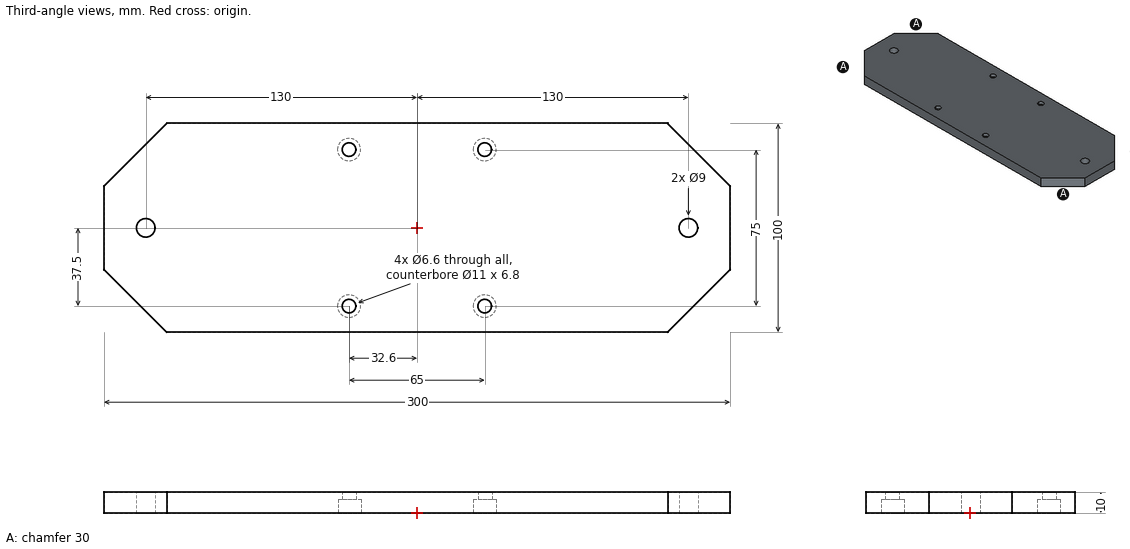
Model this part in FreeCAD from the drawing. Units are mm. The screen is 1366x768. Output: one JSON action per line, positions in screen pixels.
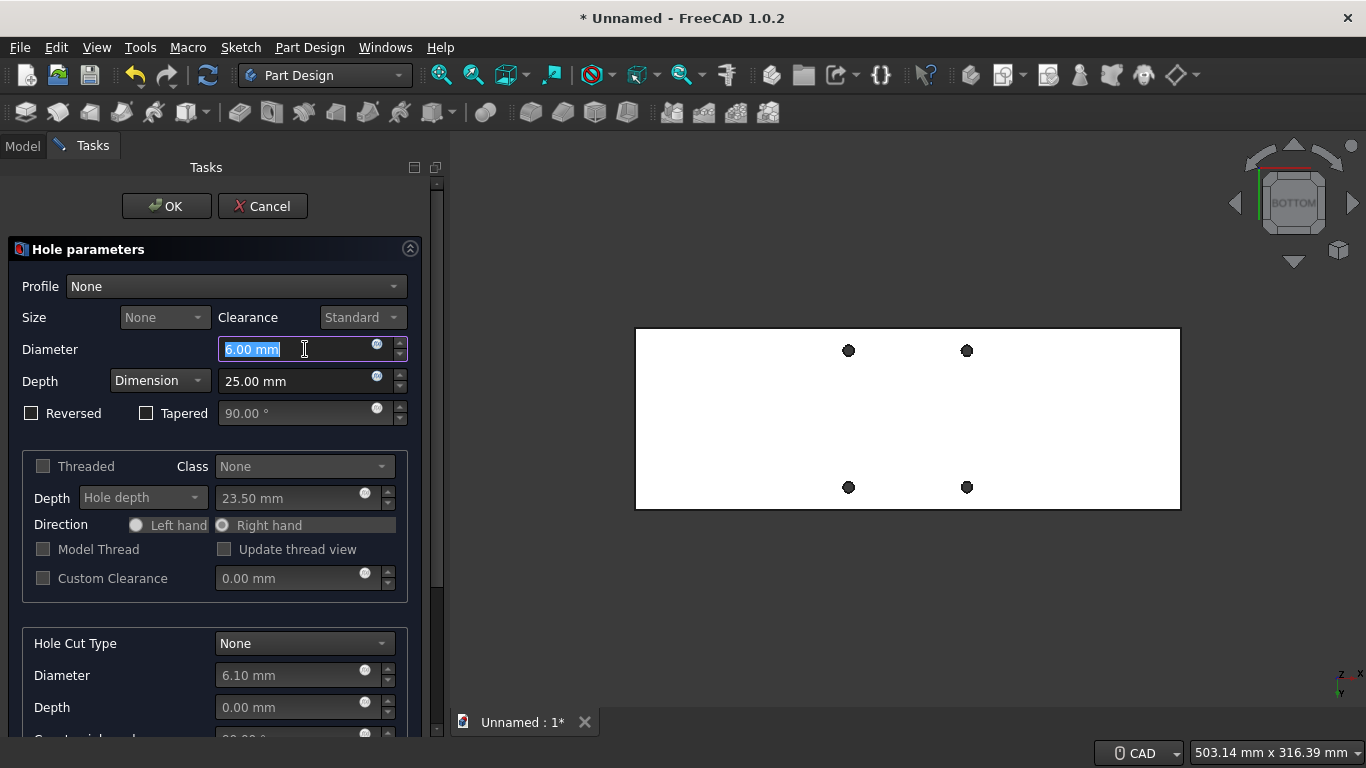
{"action": "type", "text": "6.6"}
{"action": "key", "text": "Tab"}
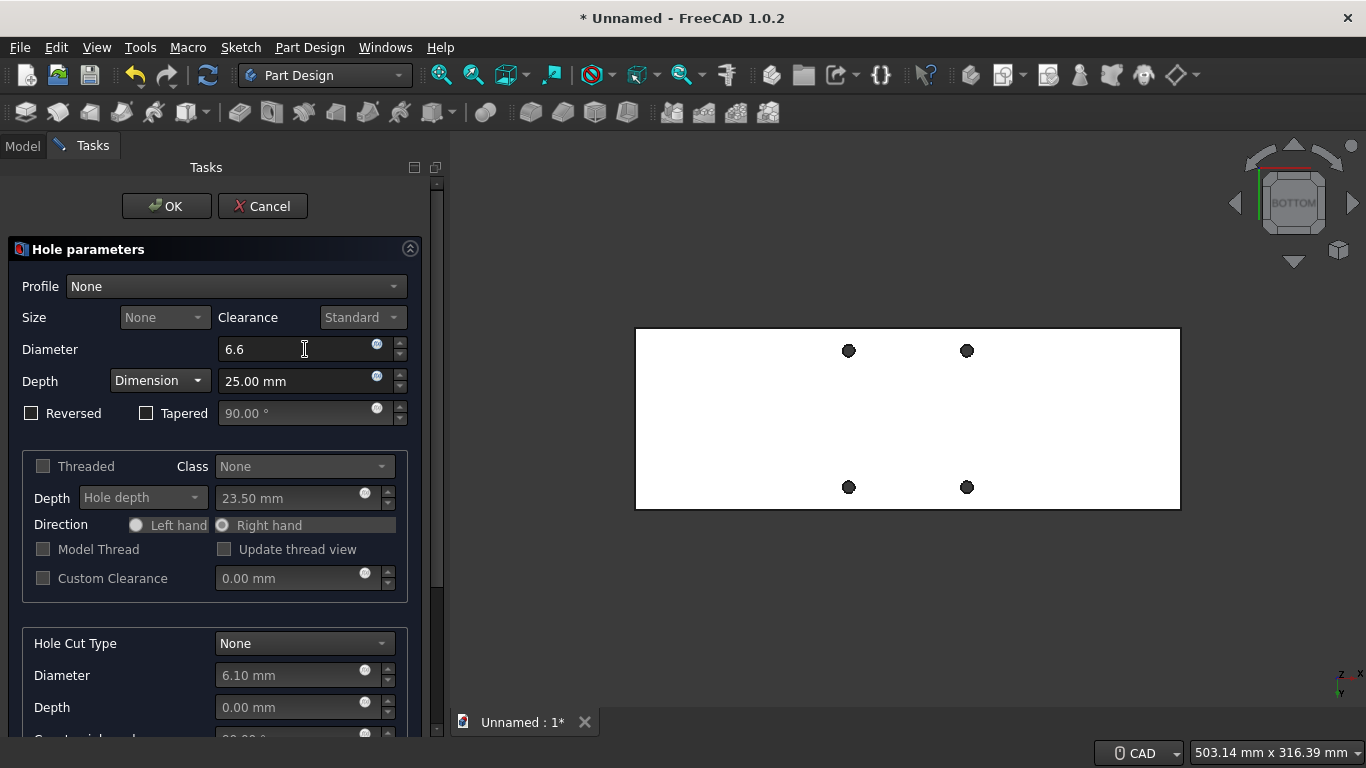
{"action": "left_click", "coordinate": [161, 380]}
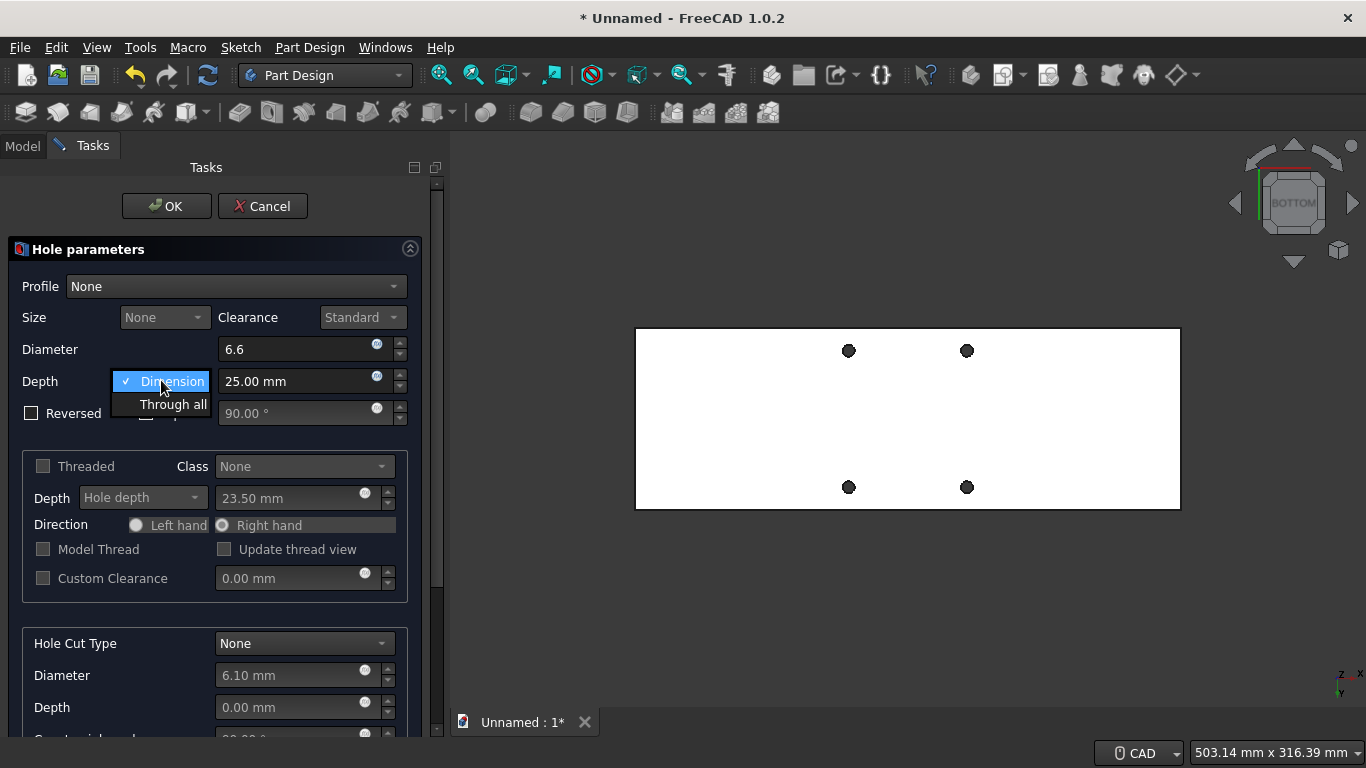
{"action": "left_click", "coordinate": [160, 404]}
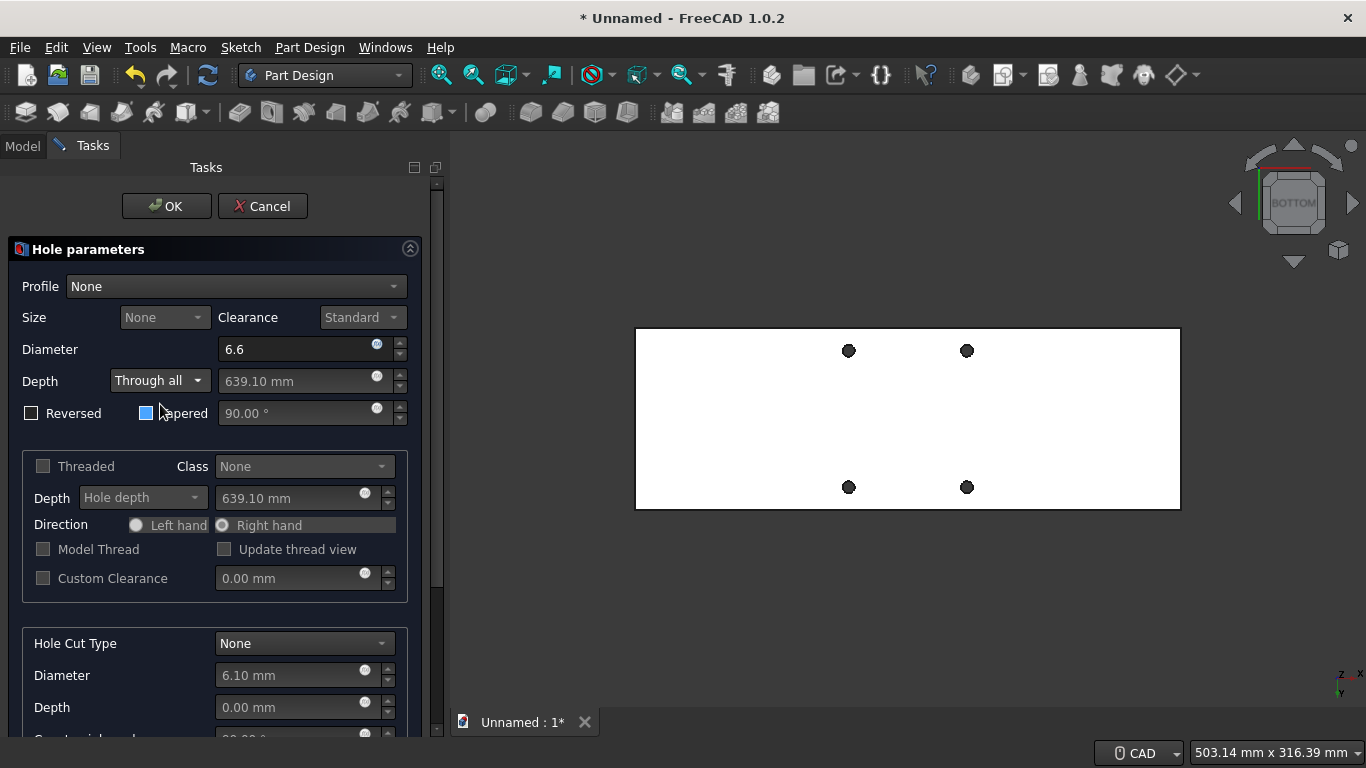
{"action": "left_click", "coordinate": [306, 644]}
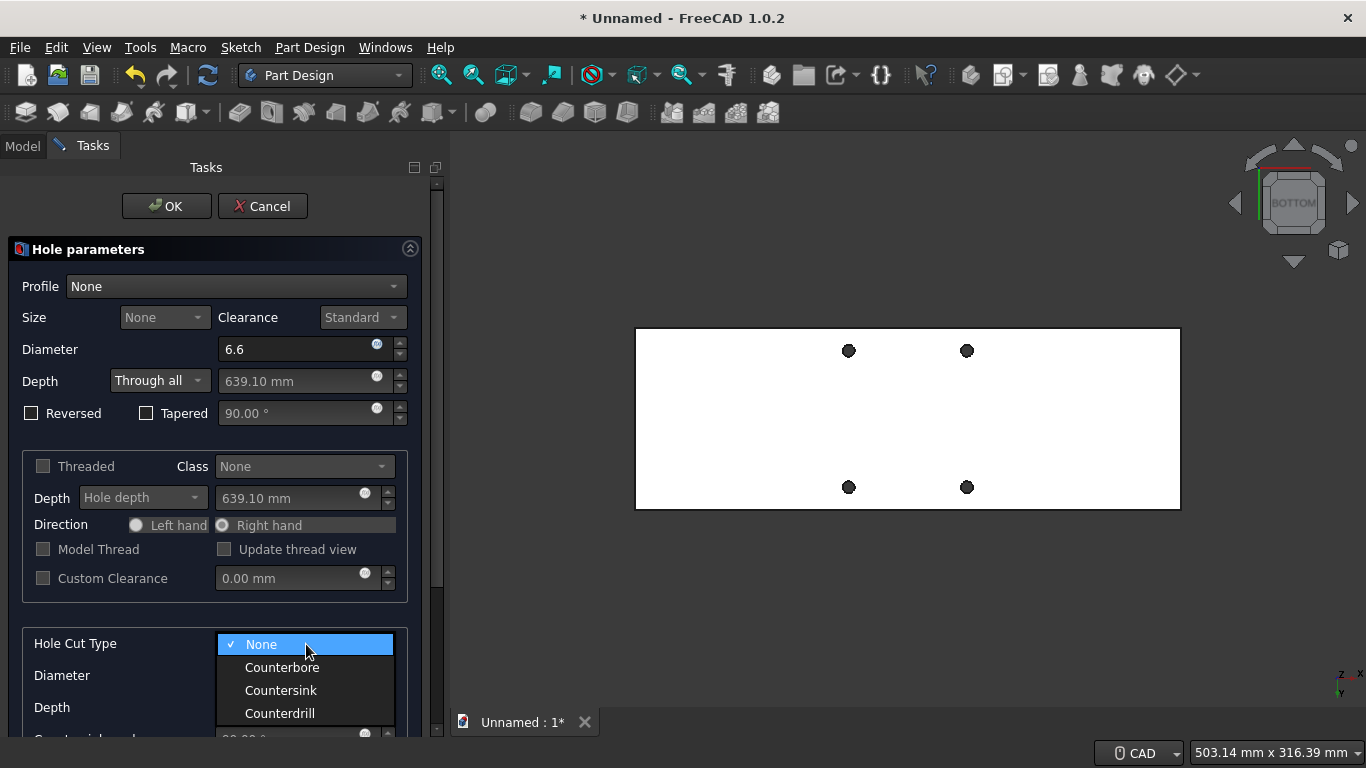
{"action": "left_click", "coordinate": [304, 668]}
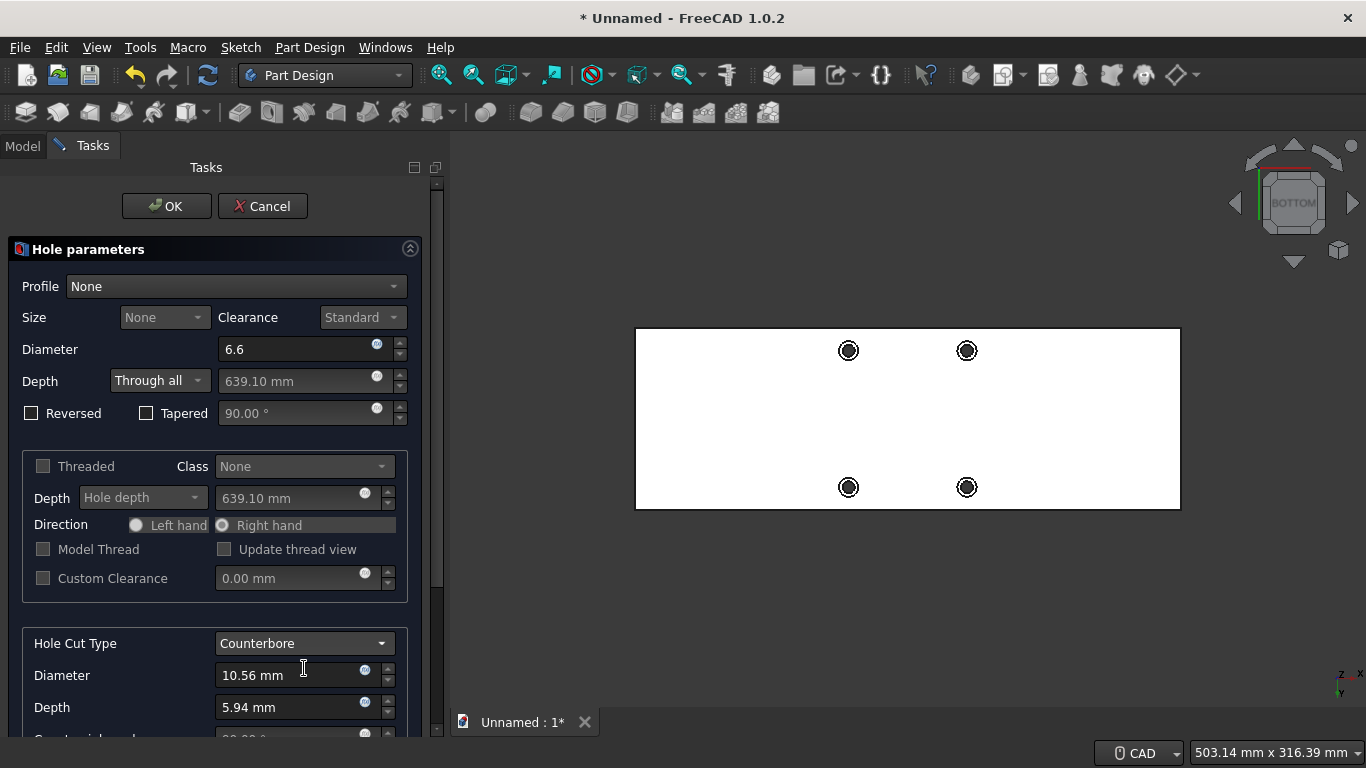
{"action": "triple_click", "coordinate": [298, 675]}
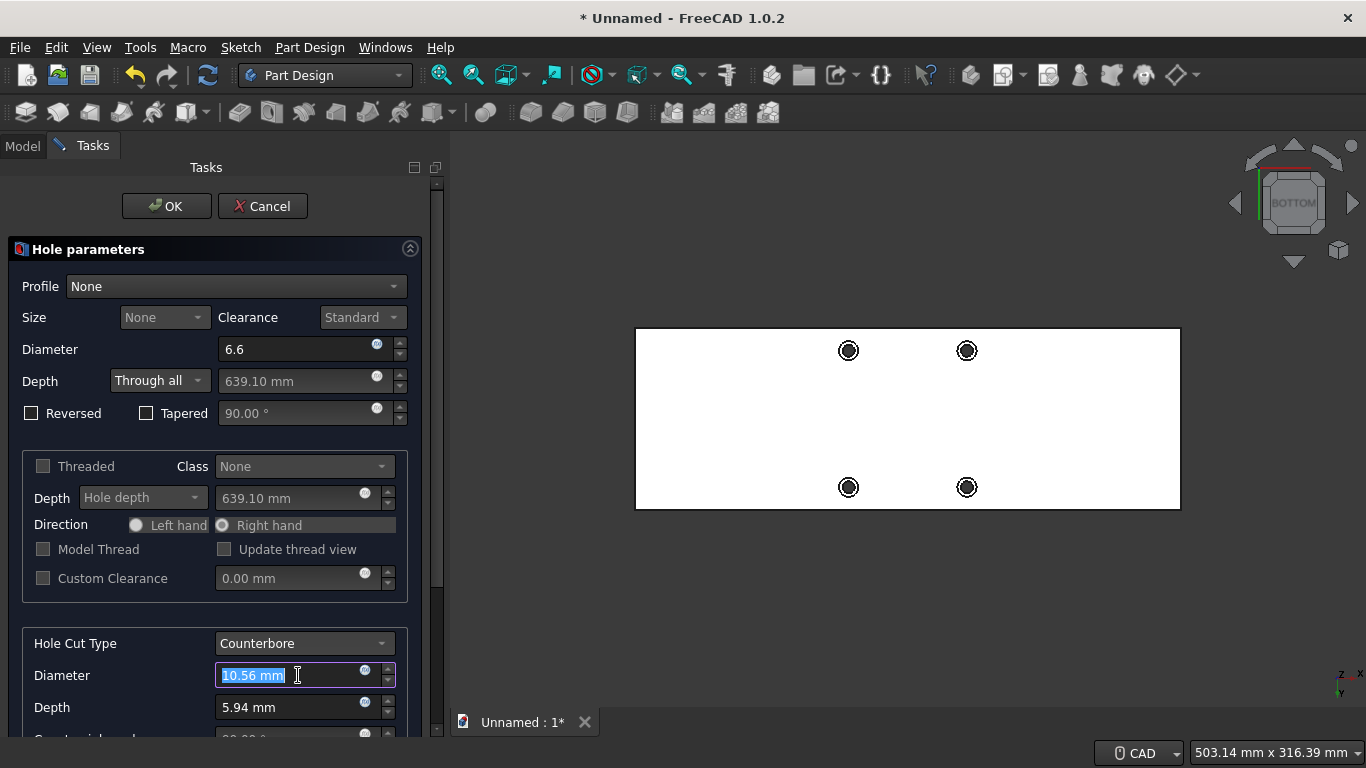
{"action": "type", "text": "11"}
{"action": "key", "text": "Tab"}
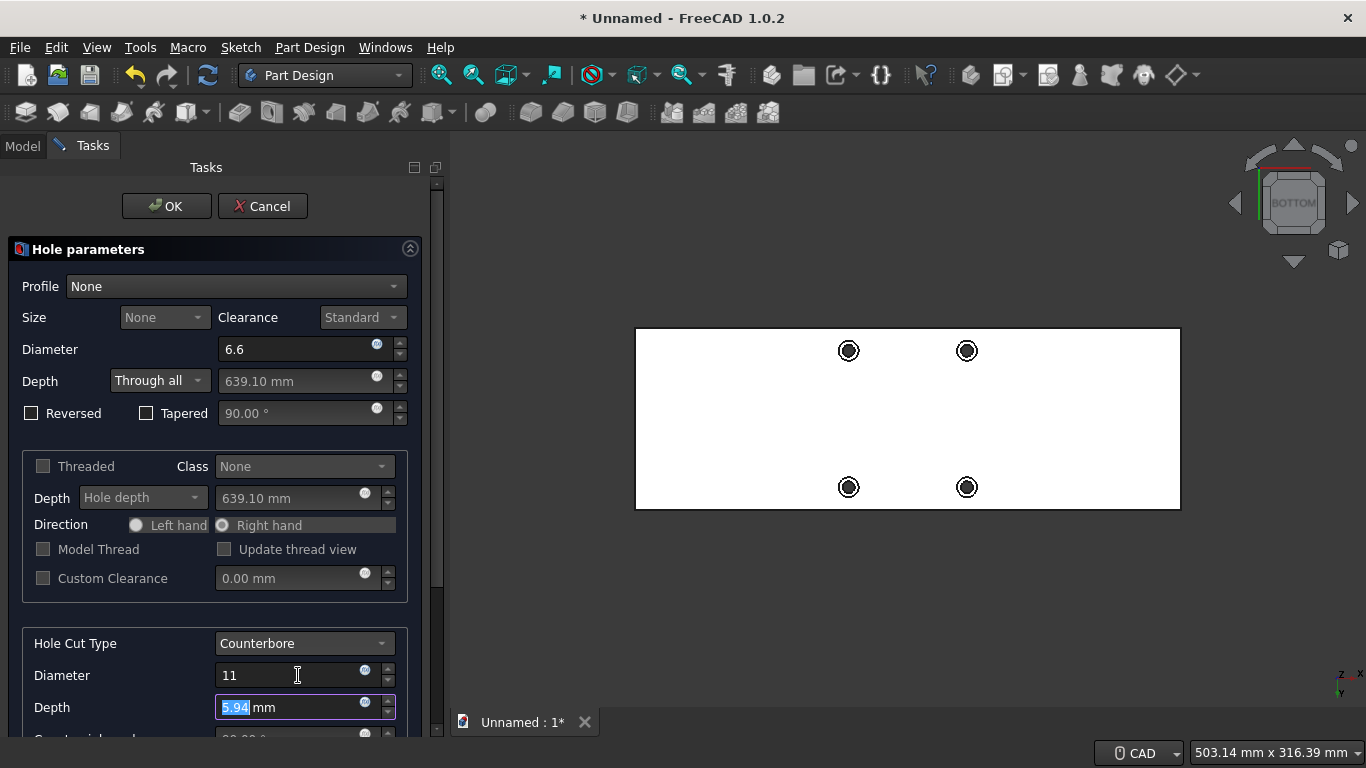
{"action": "type", "text": "6.8"}
{"action": "key", "text": "Tab"}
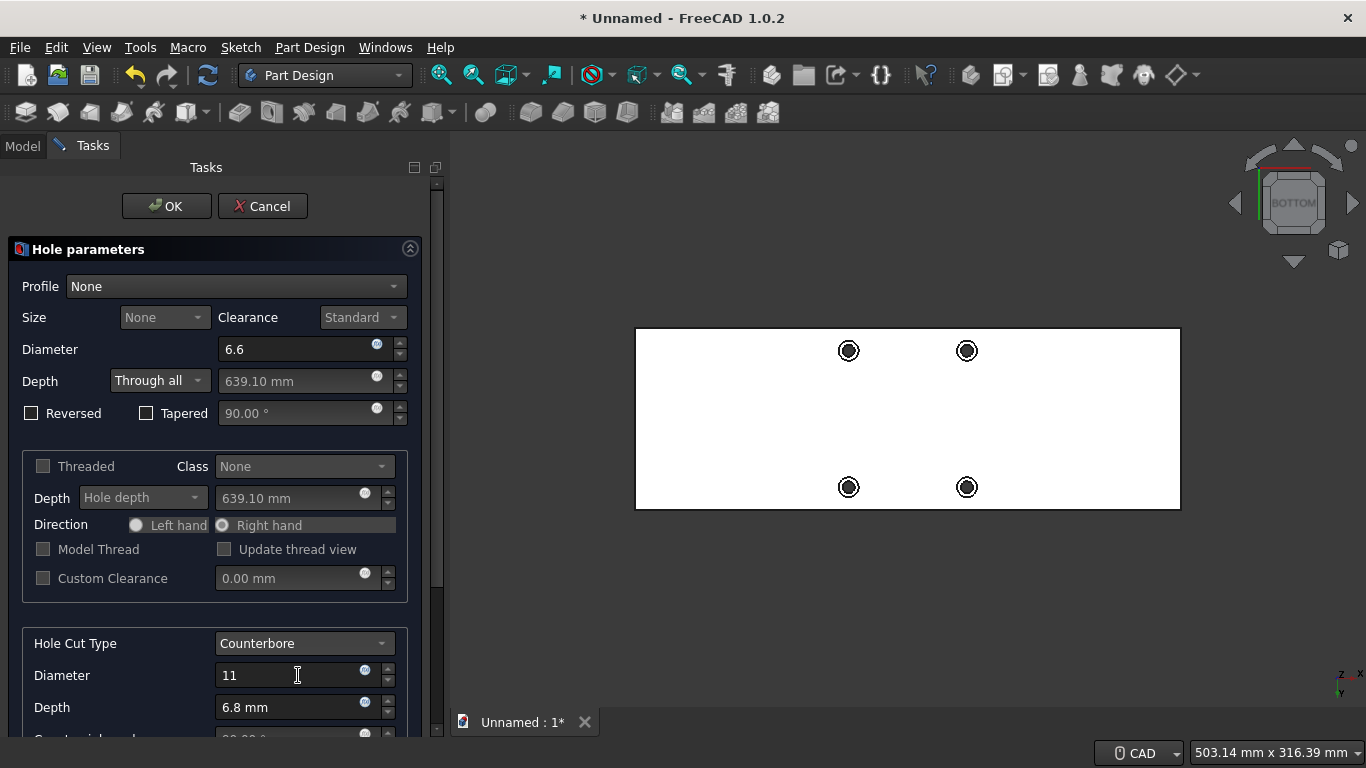
{"action": "left_click", "coordinate": [167, 206]}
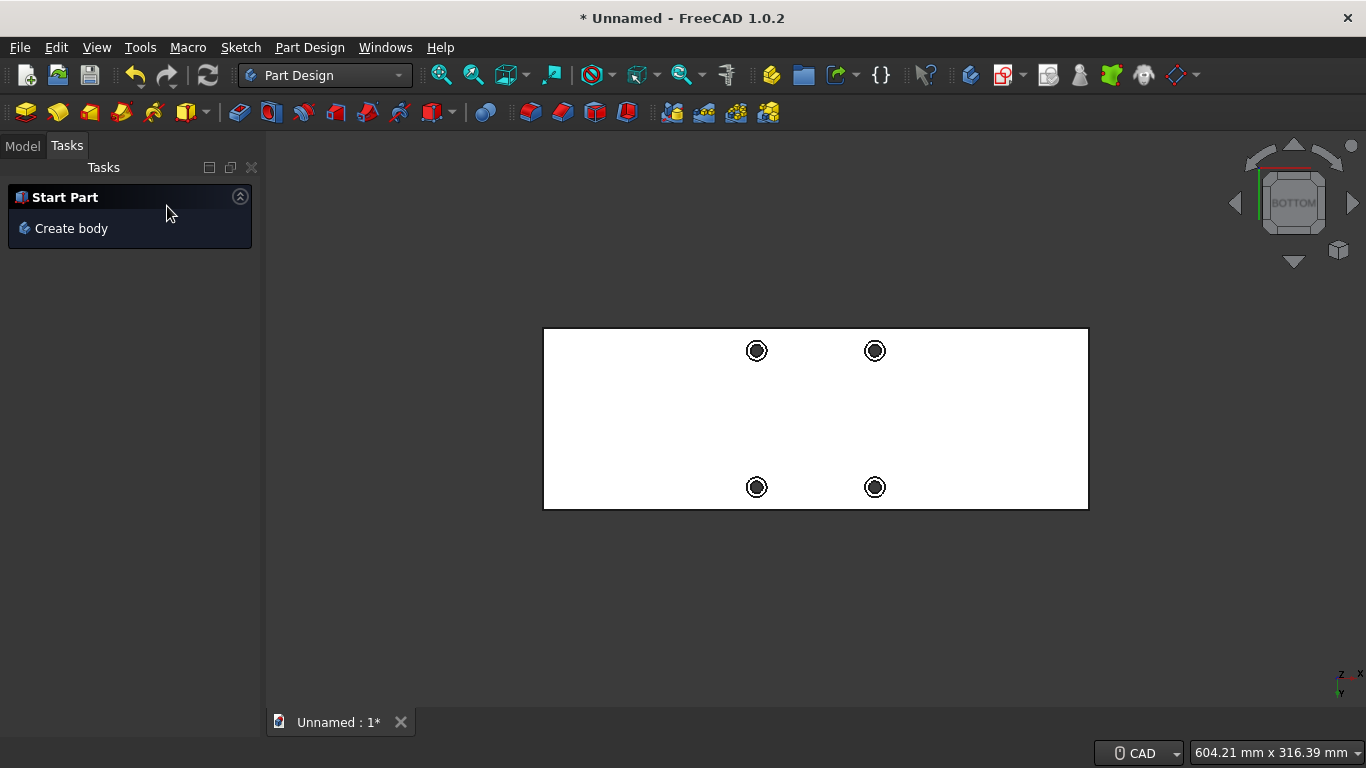
{"action": "left_click", "coordinate": [1004, 76]}